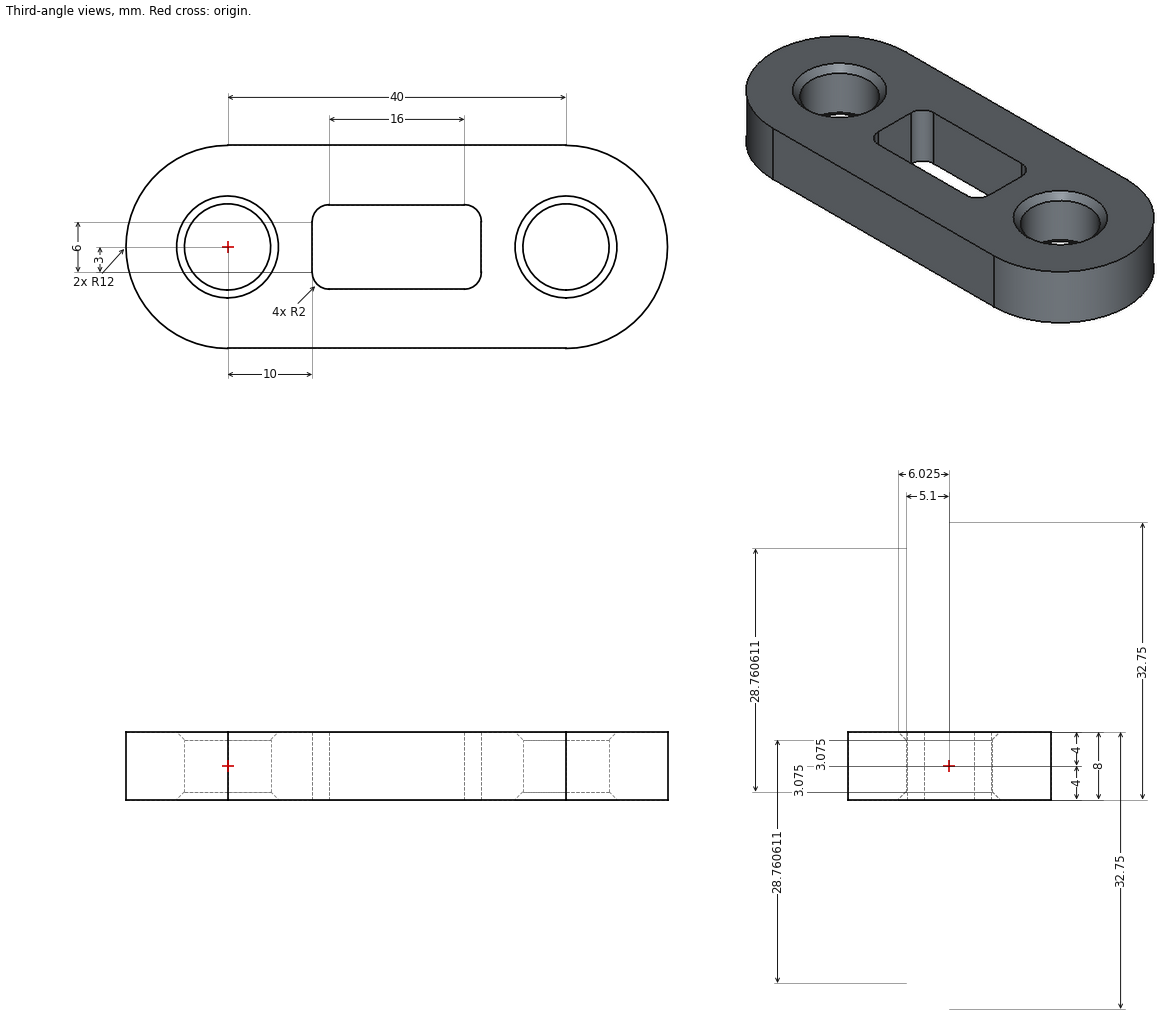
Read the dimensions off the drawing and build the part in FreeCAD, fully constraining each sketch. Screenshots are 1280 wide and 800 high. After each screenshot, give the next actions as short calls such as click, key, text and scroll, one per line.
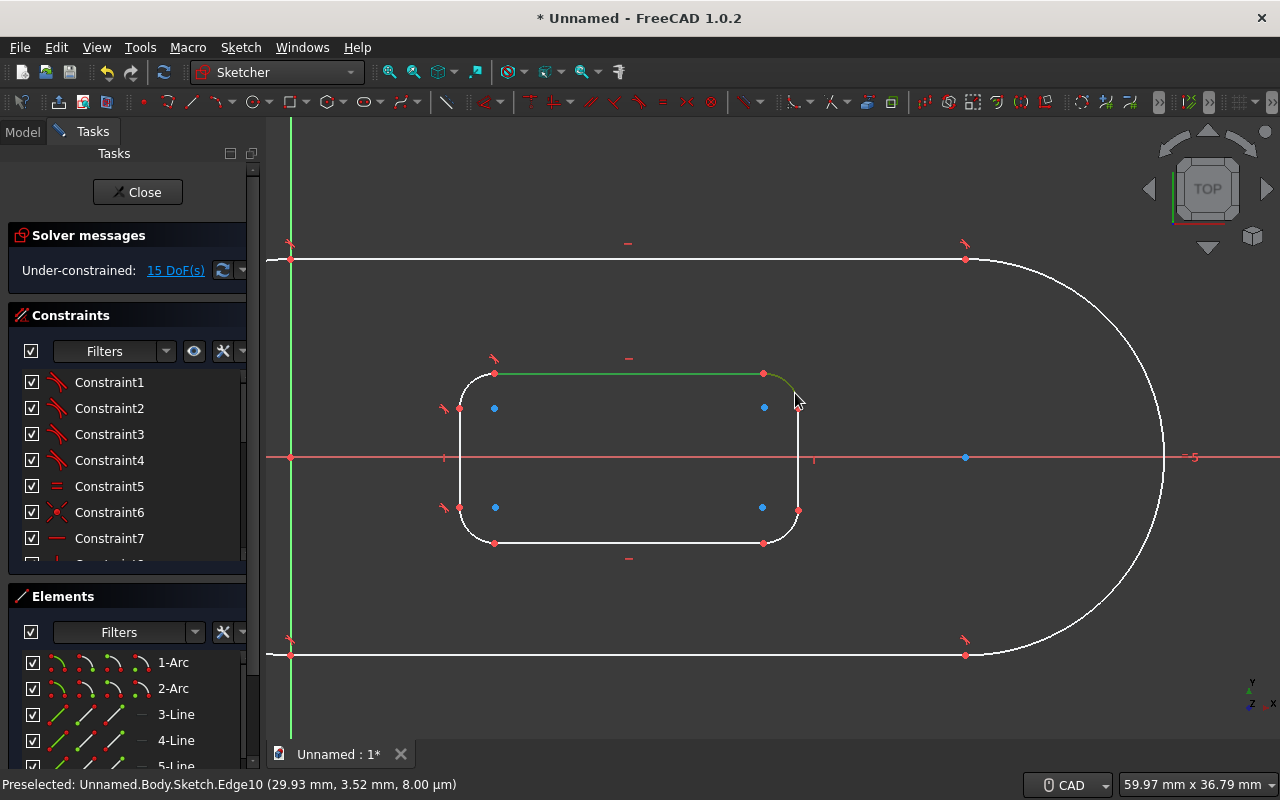
key(t)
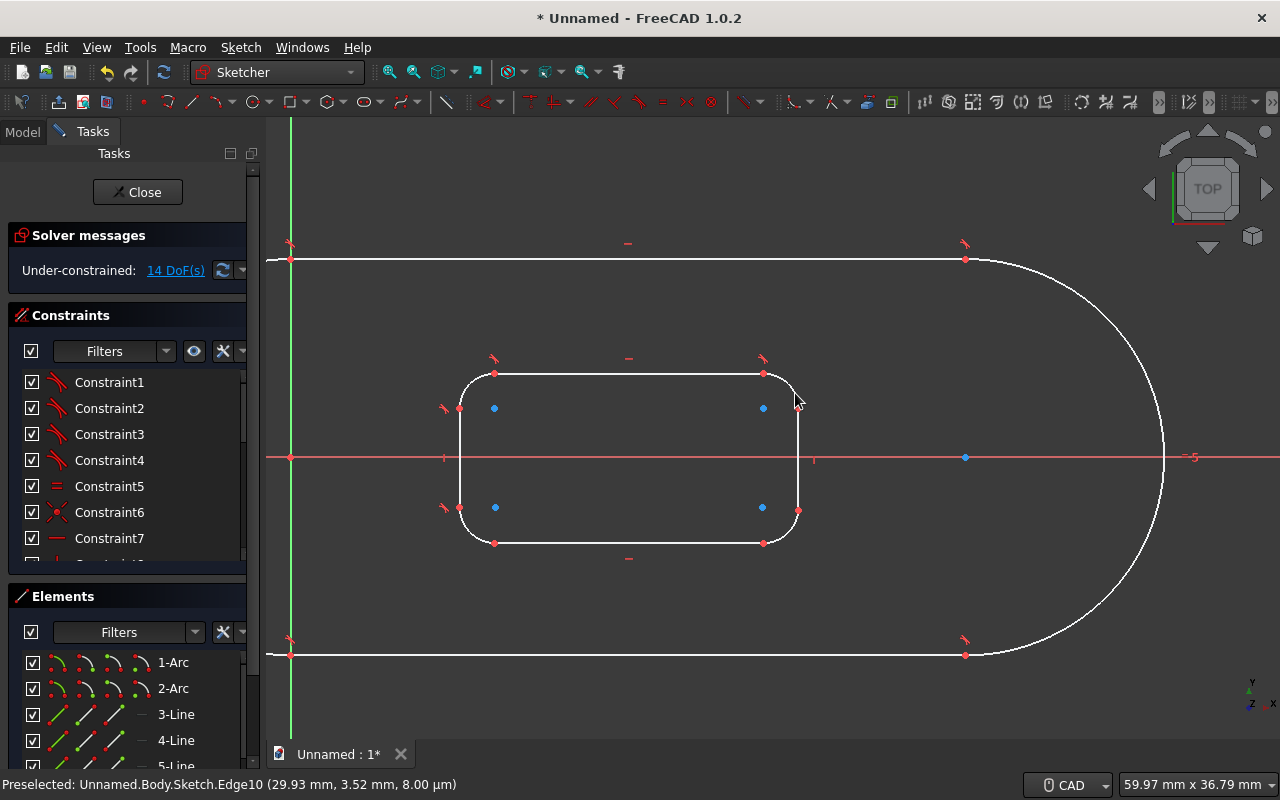
click(798, 439)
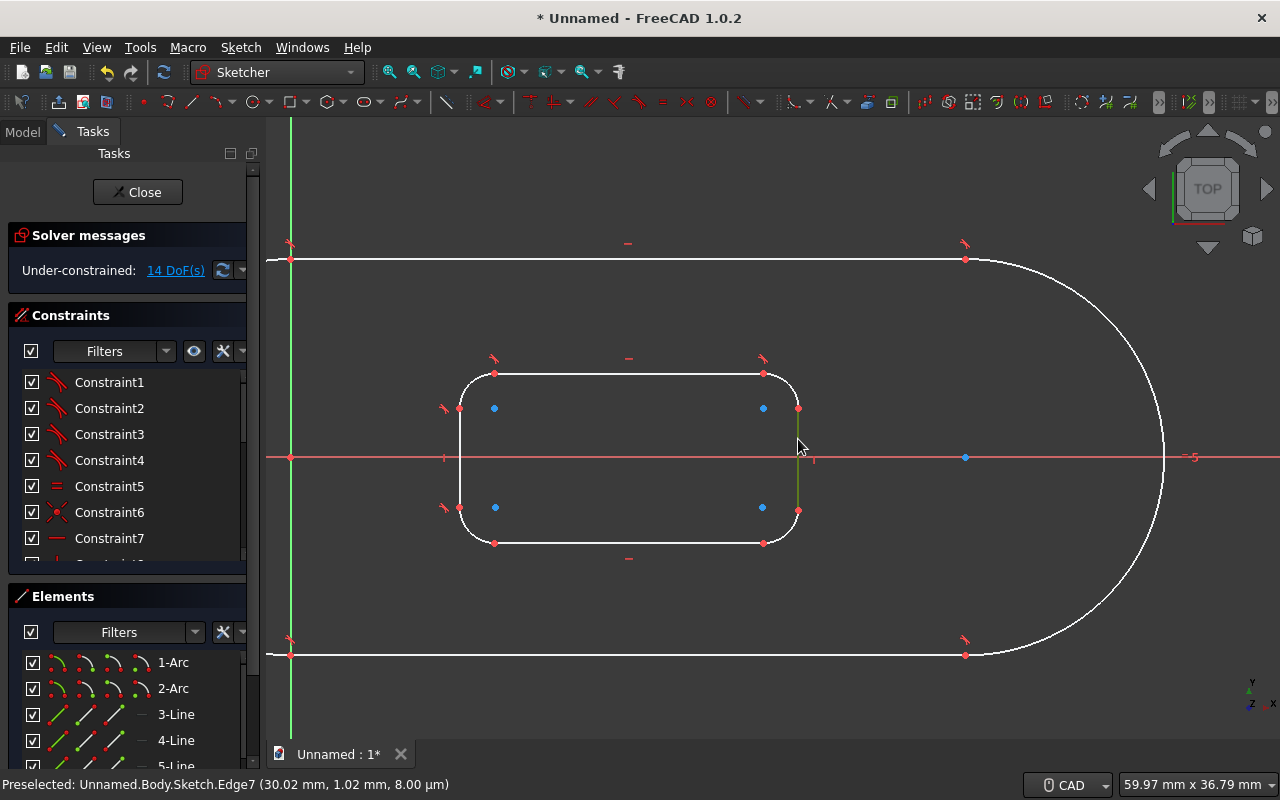
click(795, 393)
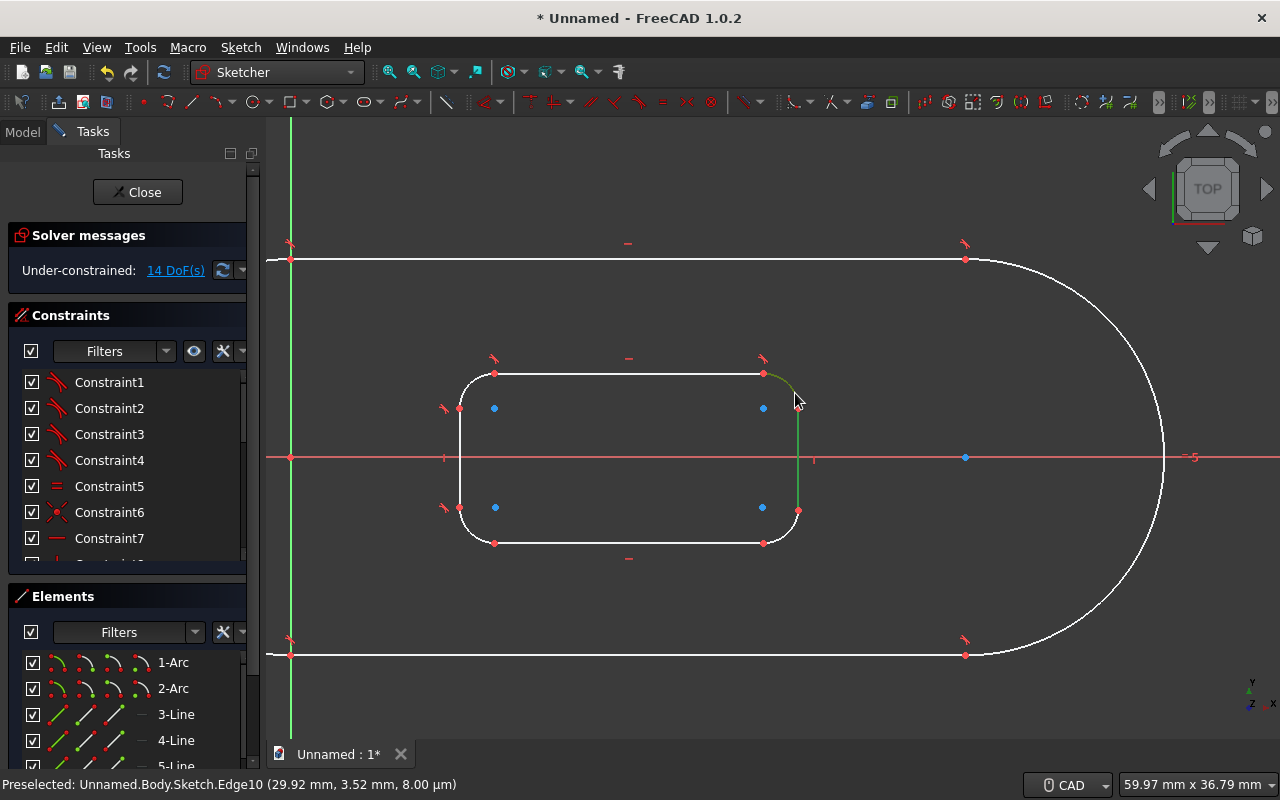
click(640, 102)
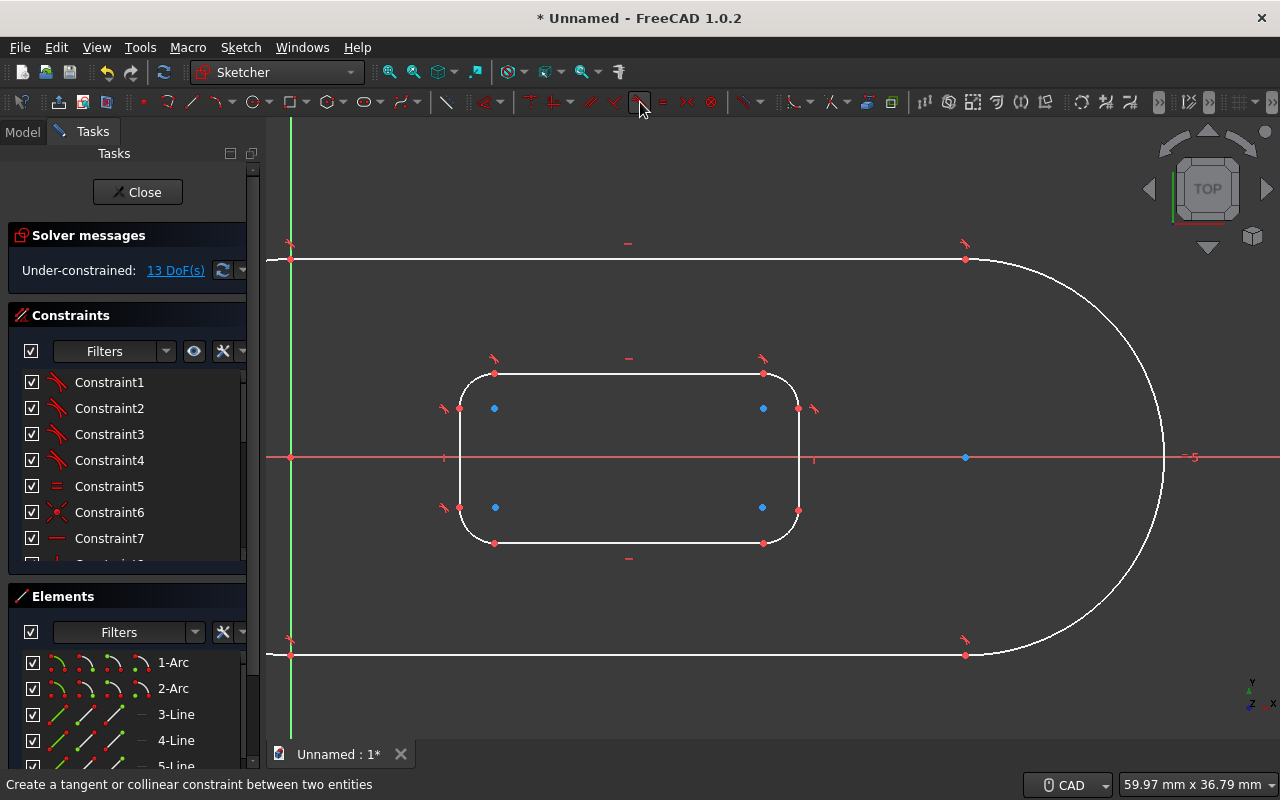
click(799, 439)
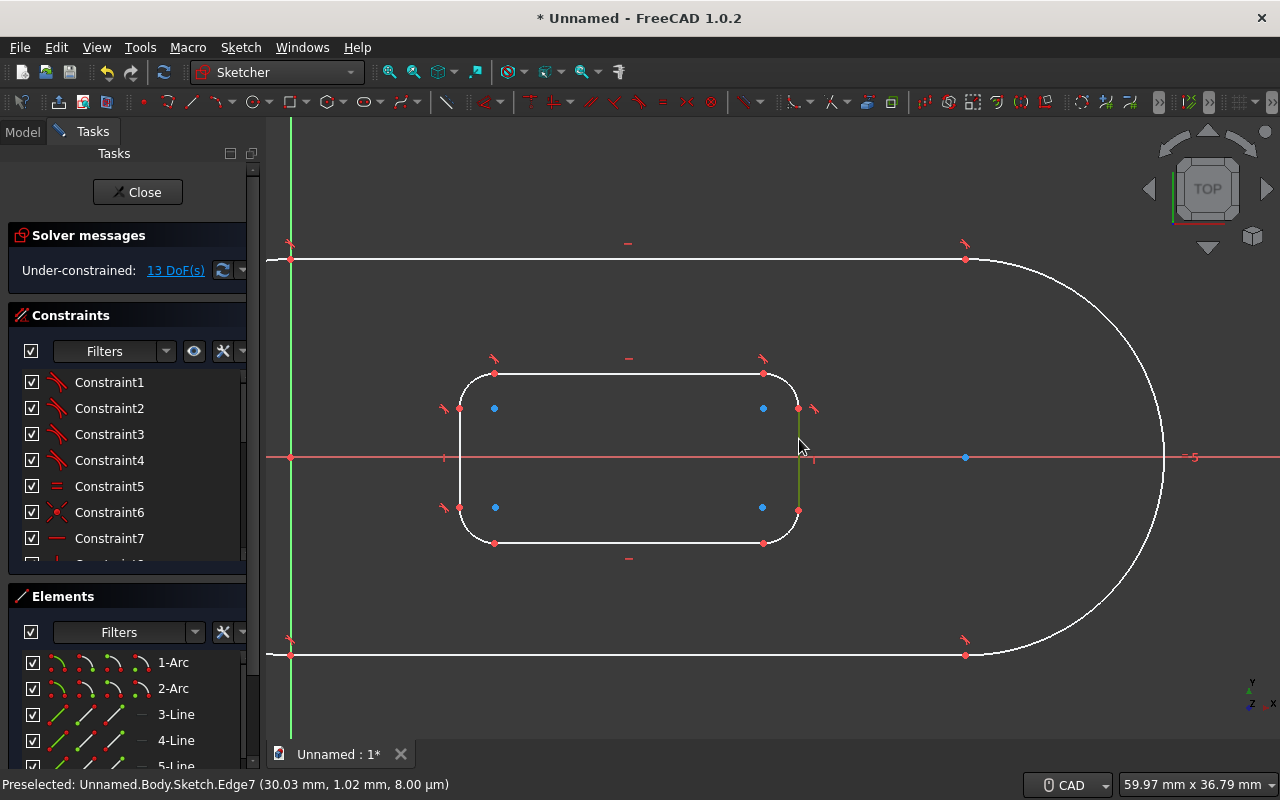
click(779, 539)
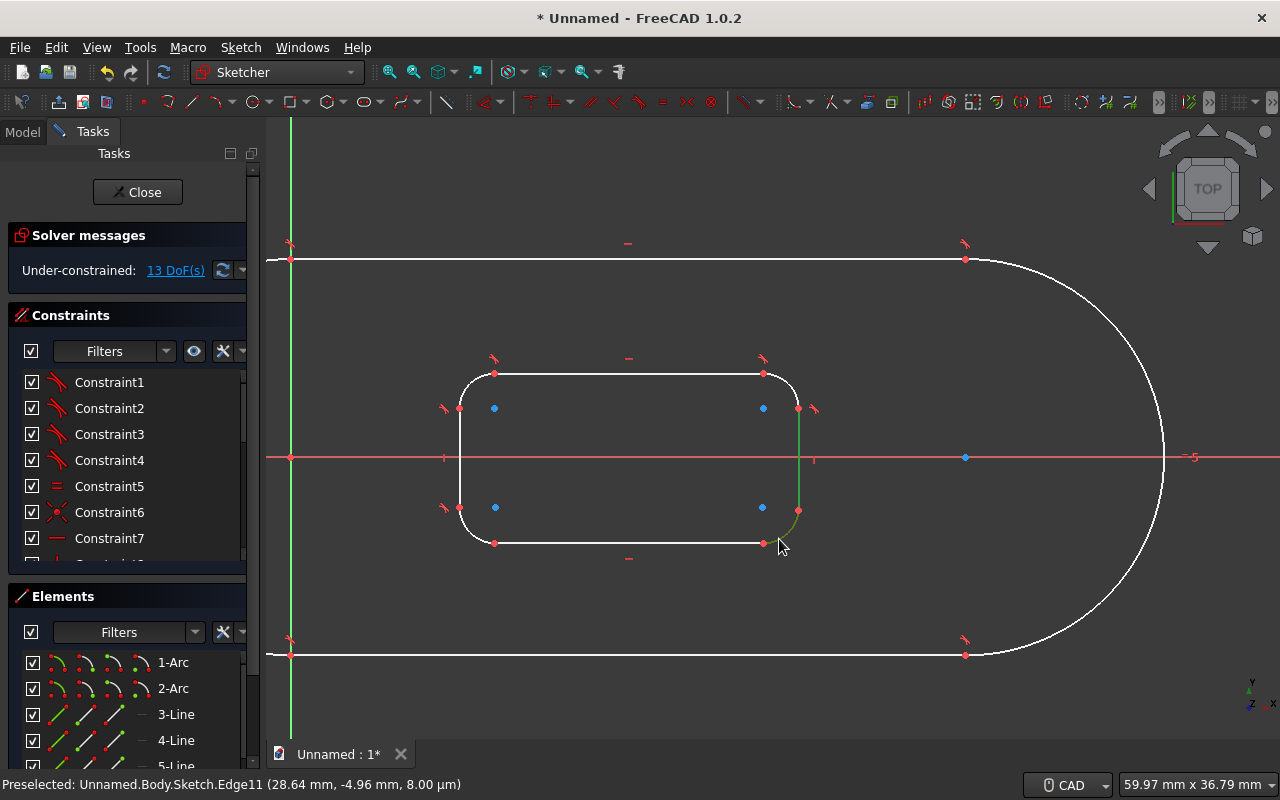
key(t)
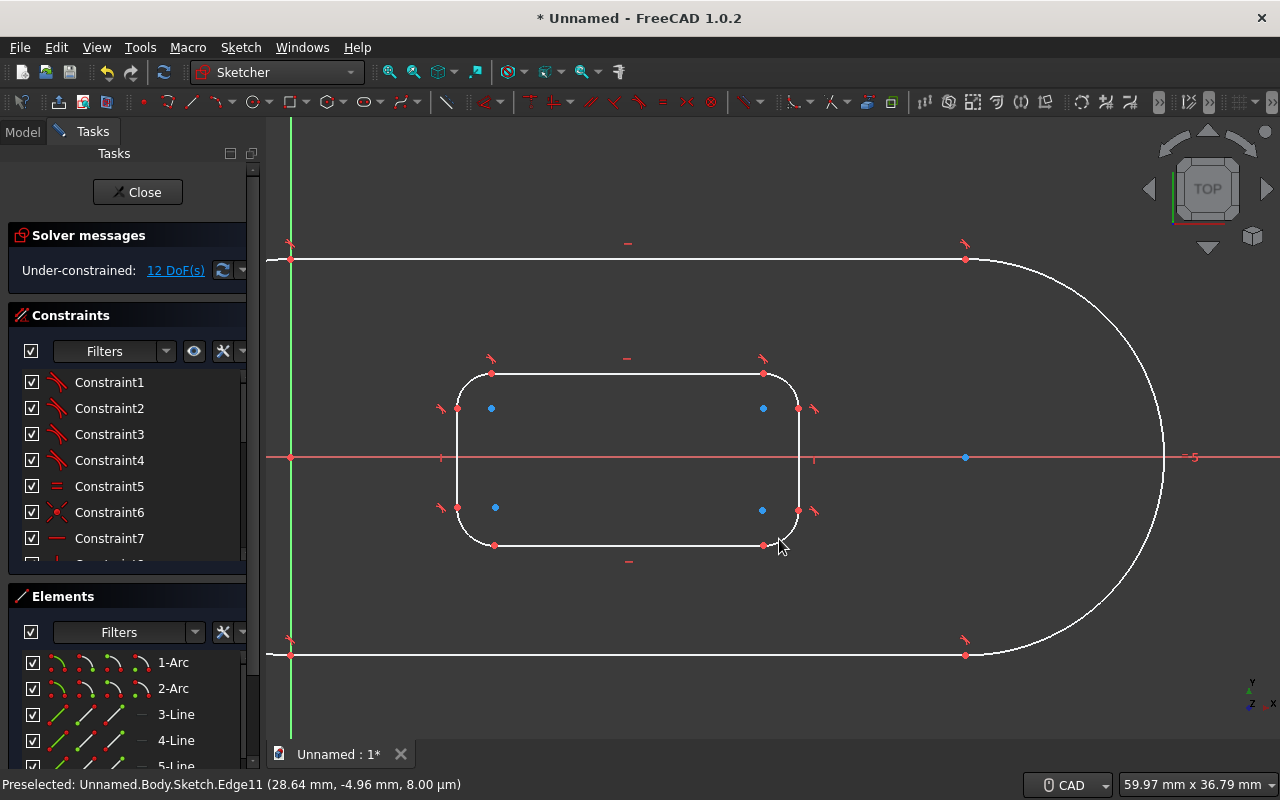
click(683, 546)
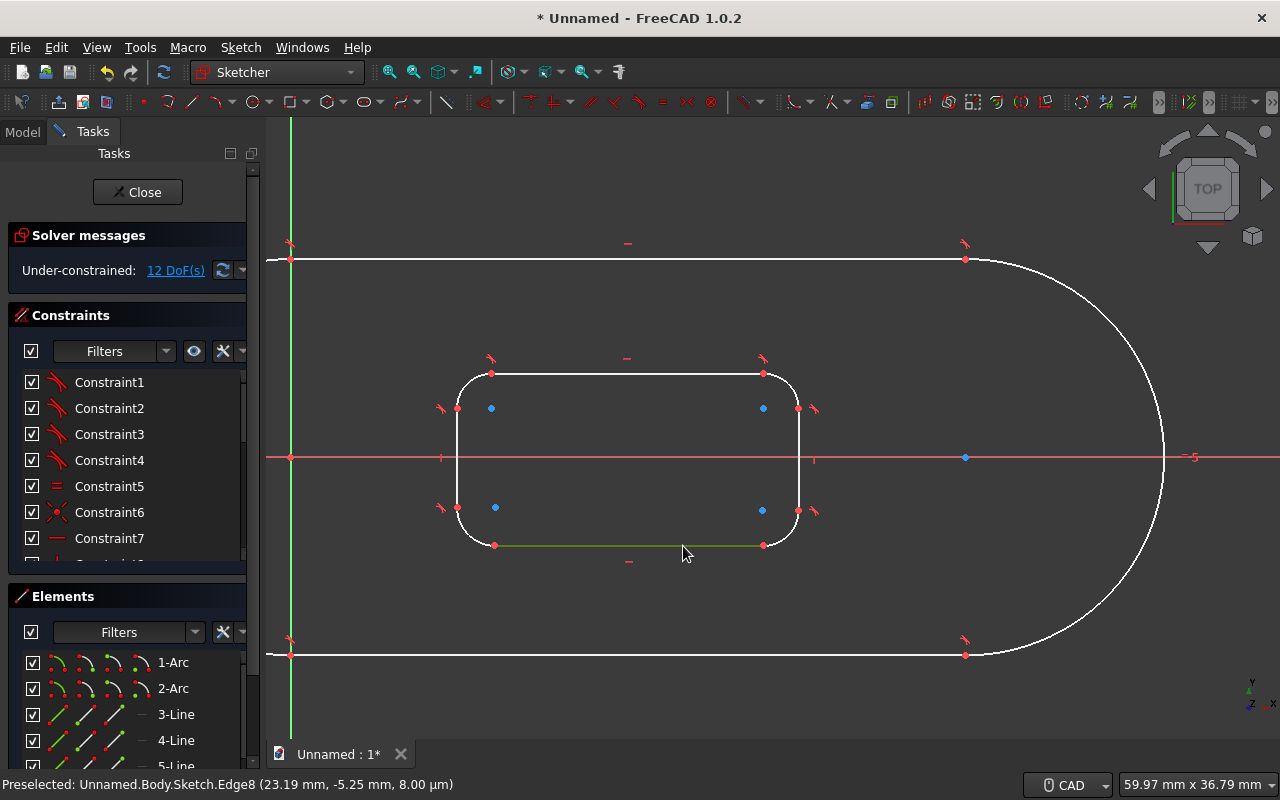
click(780, 542)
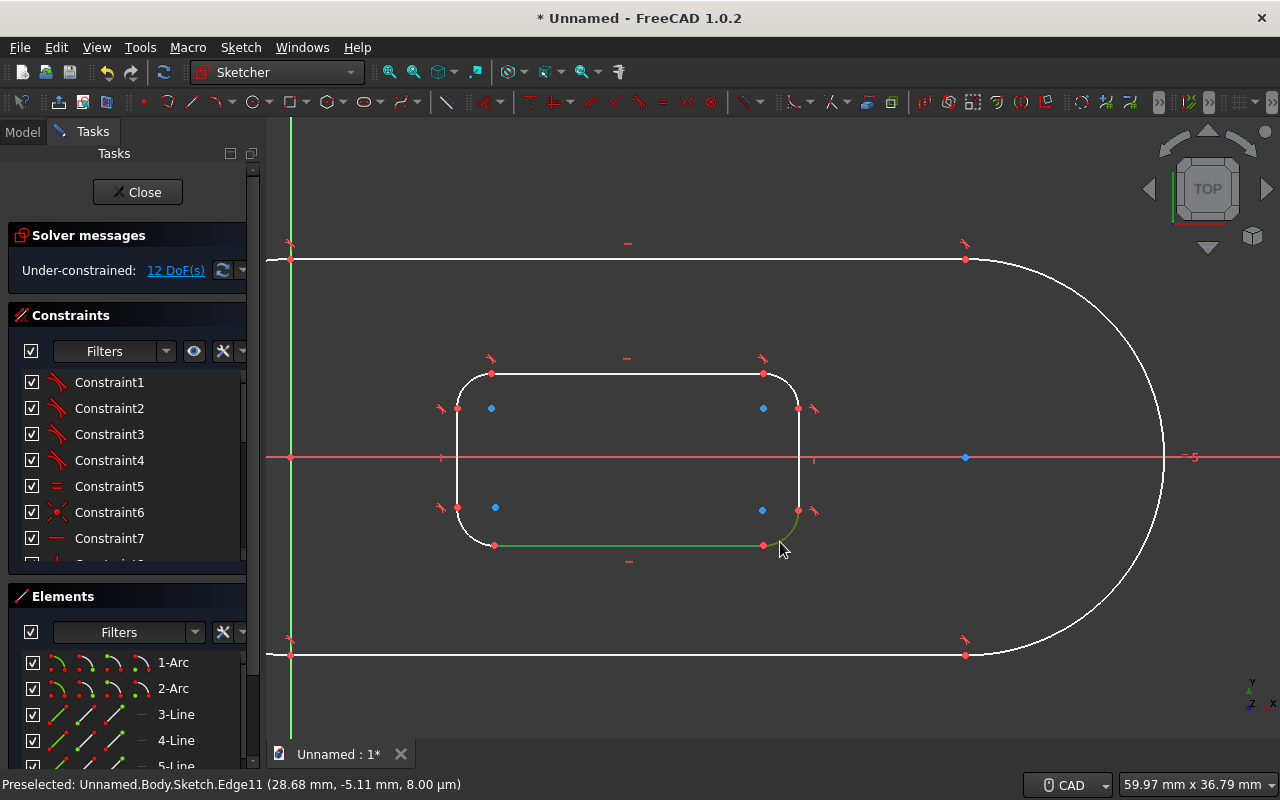
key(t)